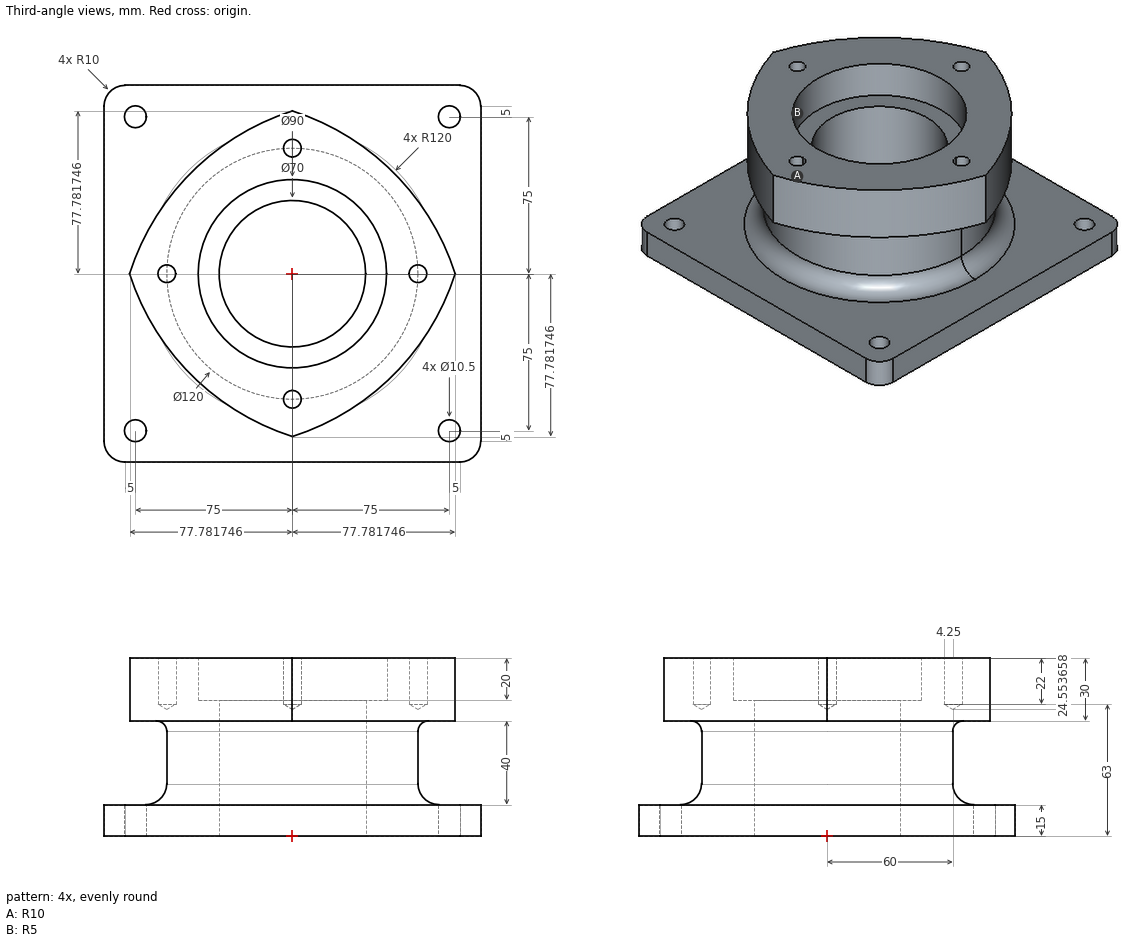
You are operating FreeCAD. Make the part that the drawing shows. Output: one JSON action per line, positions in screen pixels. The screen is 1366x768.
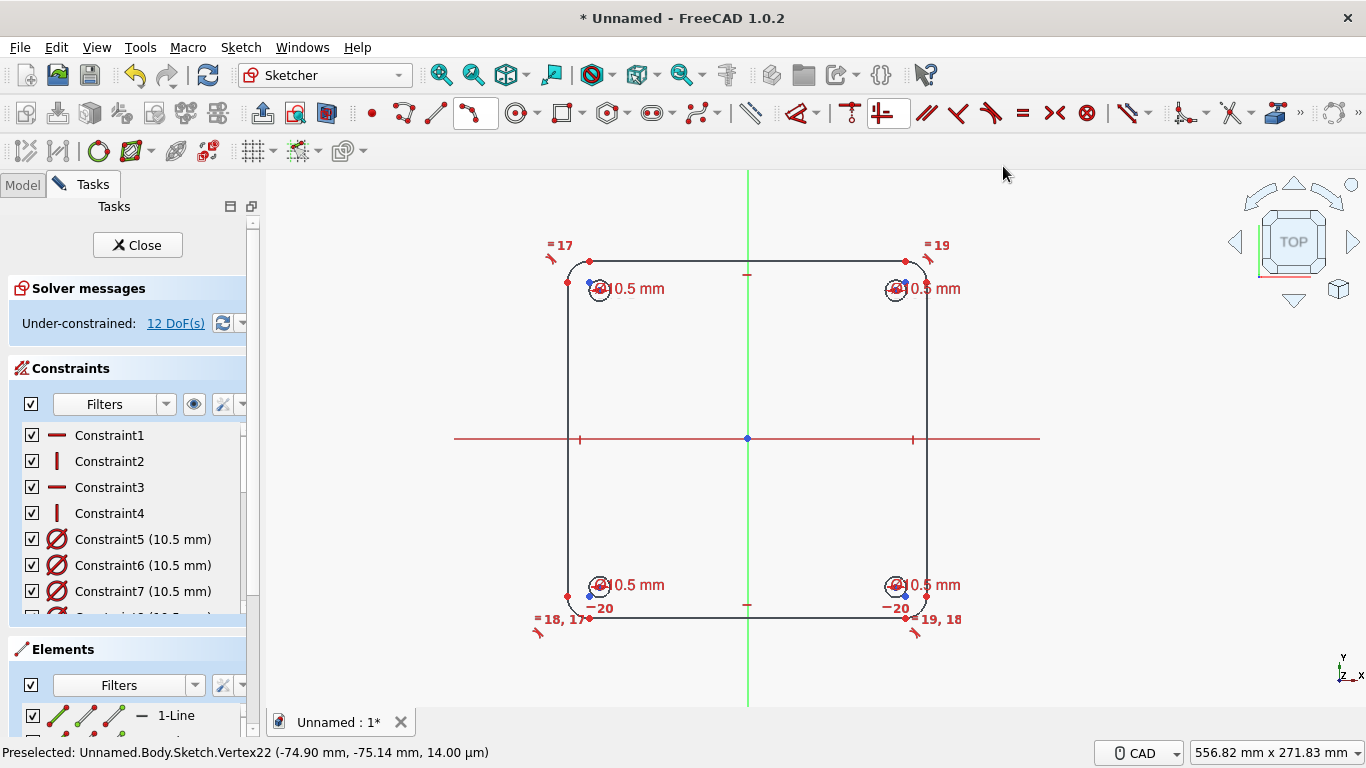
{"action": "left_click", "coordinate": [896, 587]}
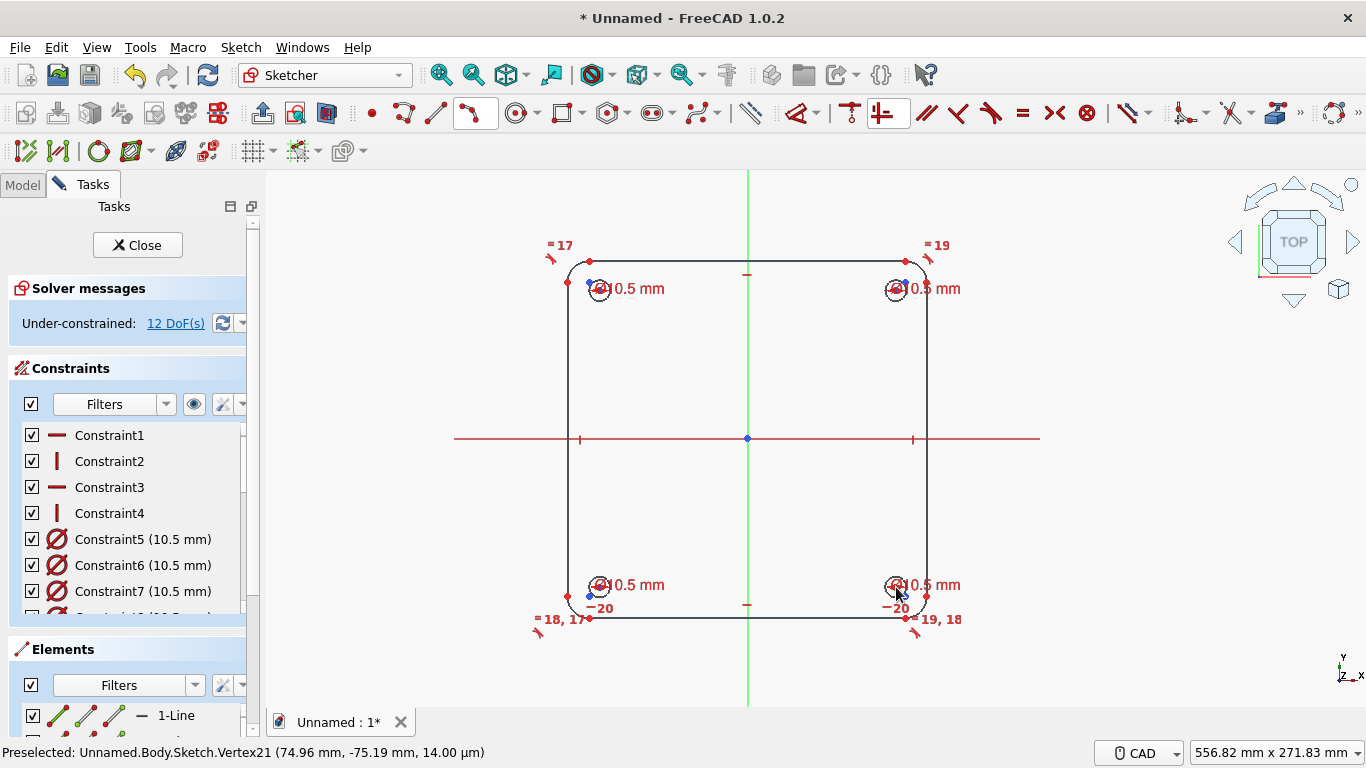
{"action": "left_click", "coordinate": [896, 291]}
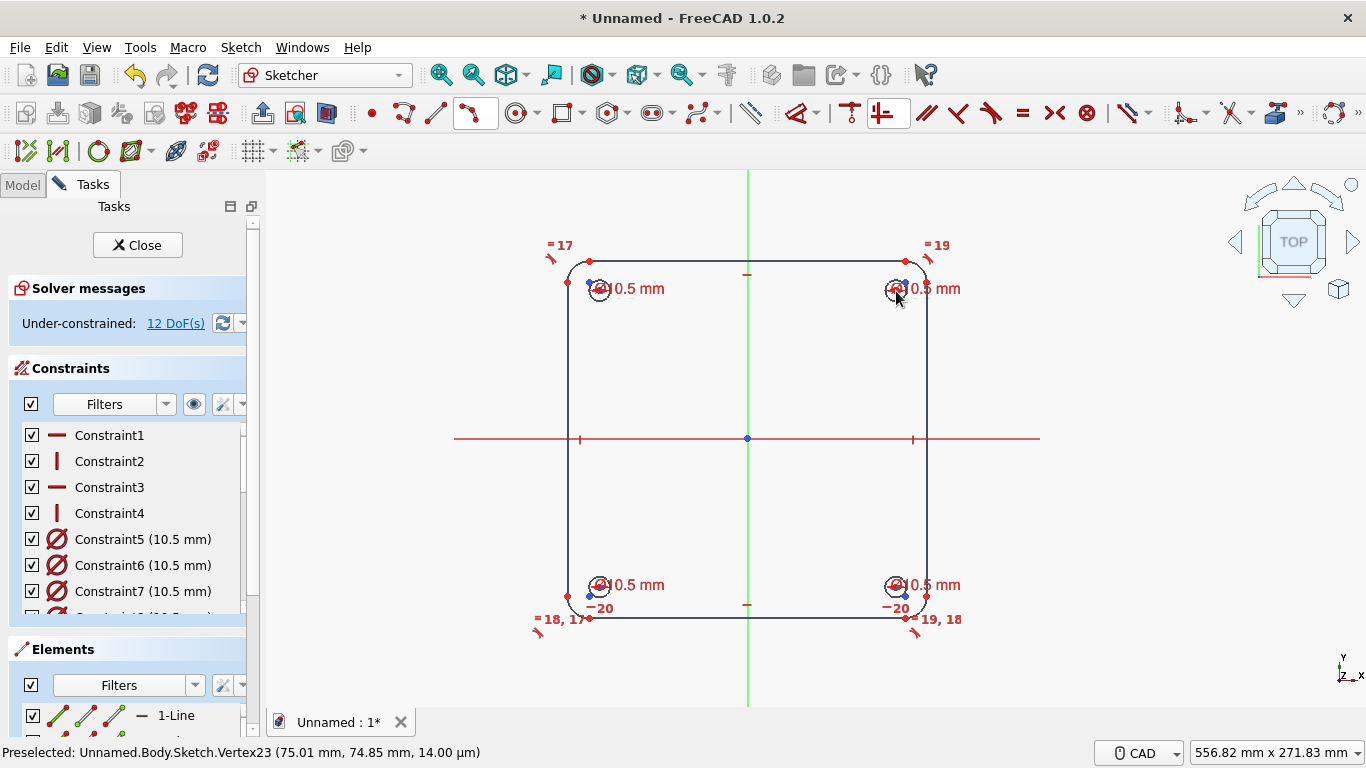
{"action": "left_click", "coordinate": [904, 114]}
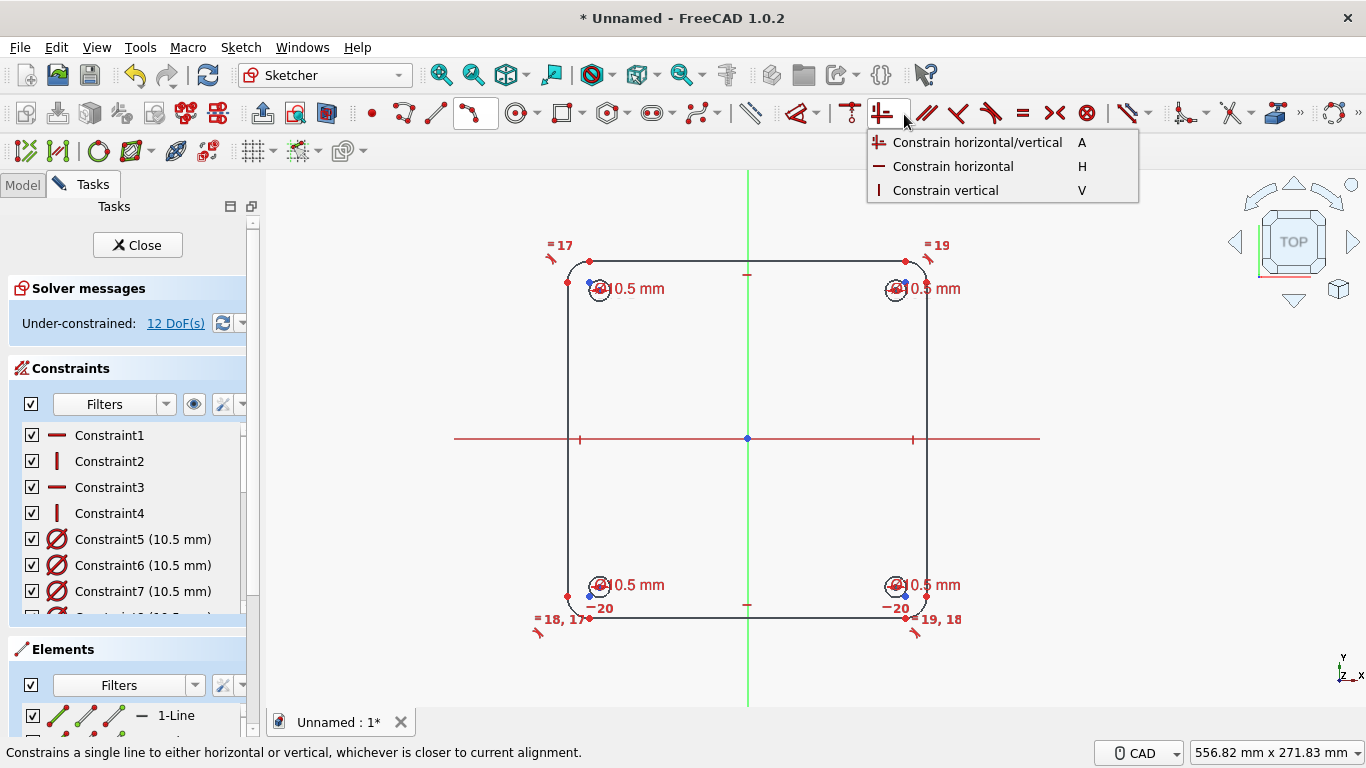
{"action": "left_click", "coordinate": [1003, 190]}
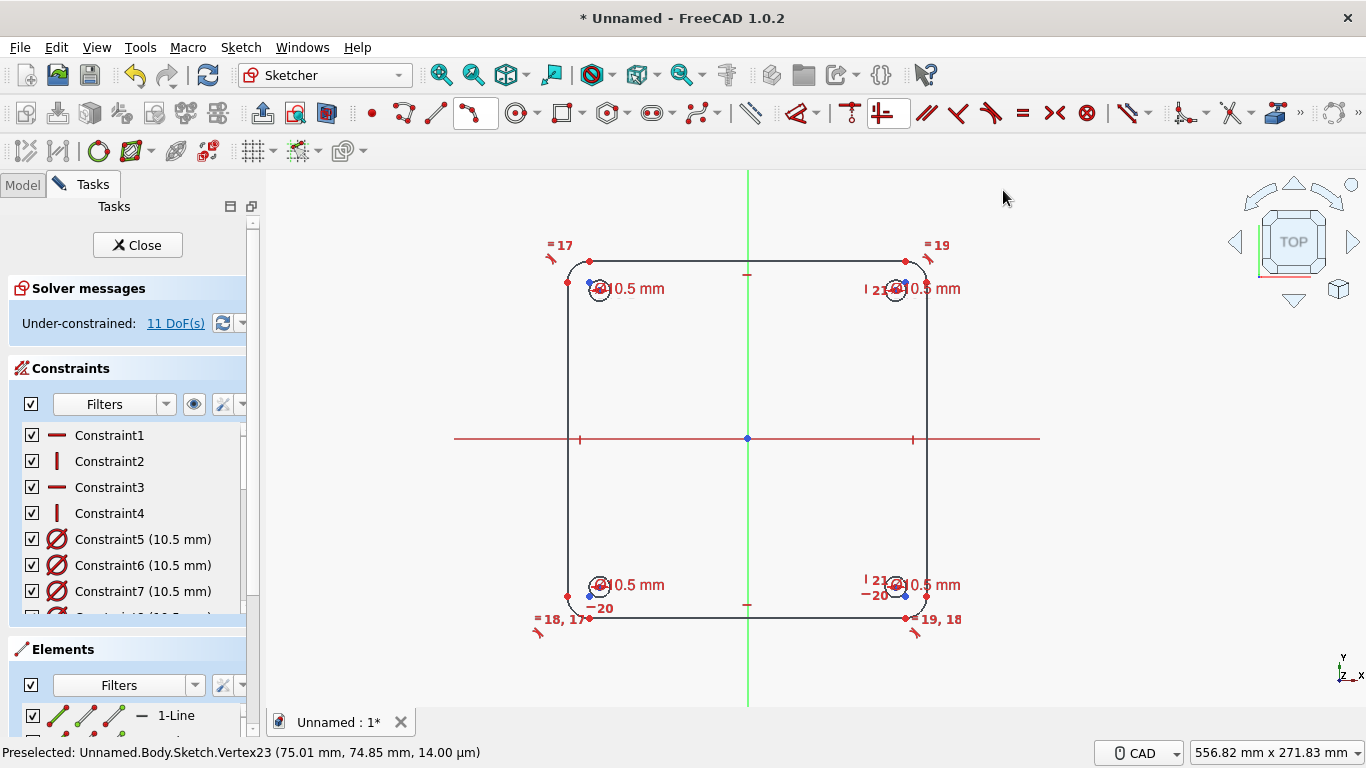
{"action": "left_click", "coordinate": [600, 587]}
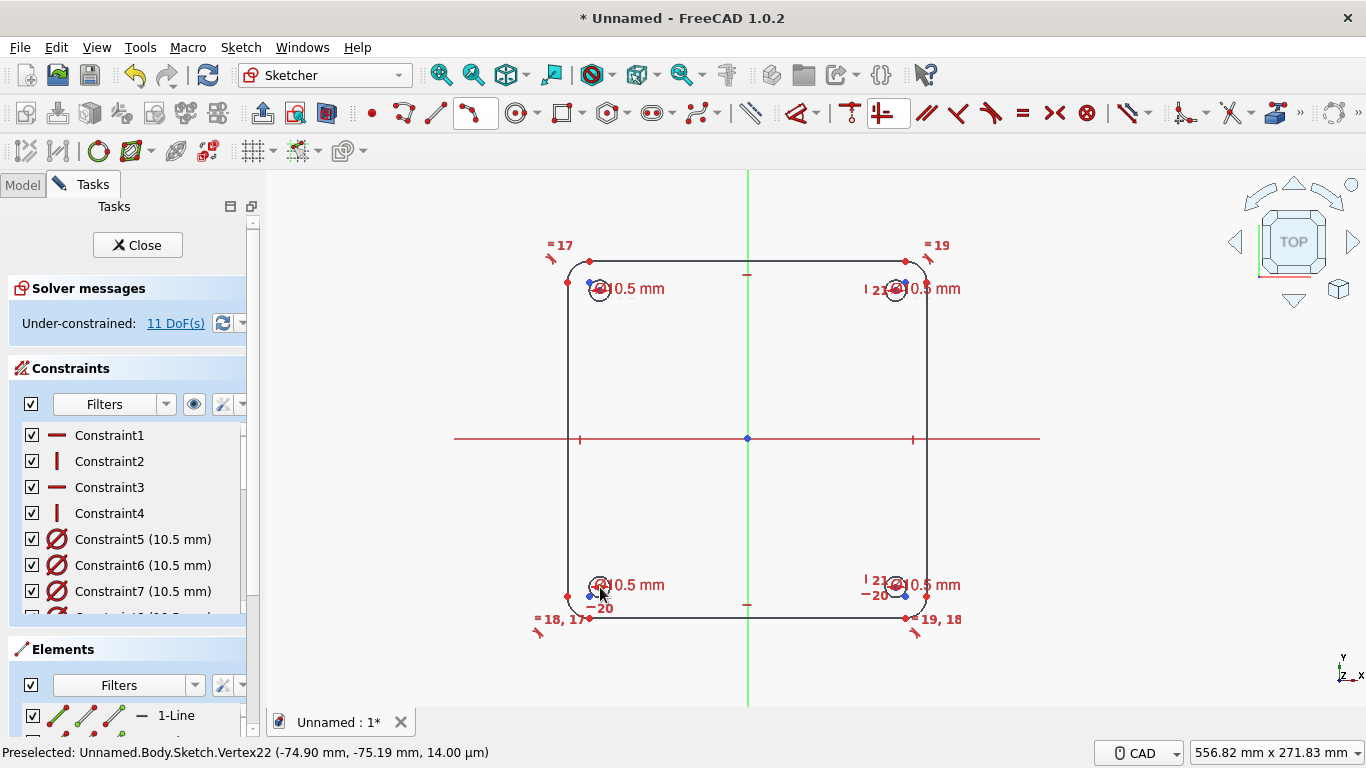
{"action": "left_click", "coordinate": [600, 291]}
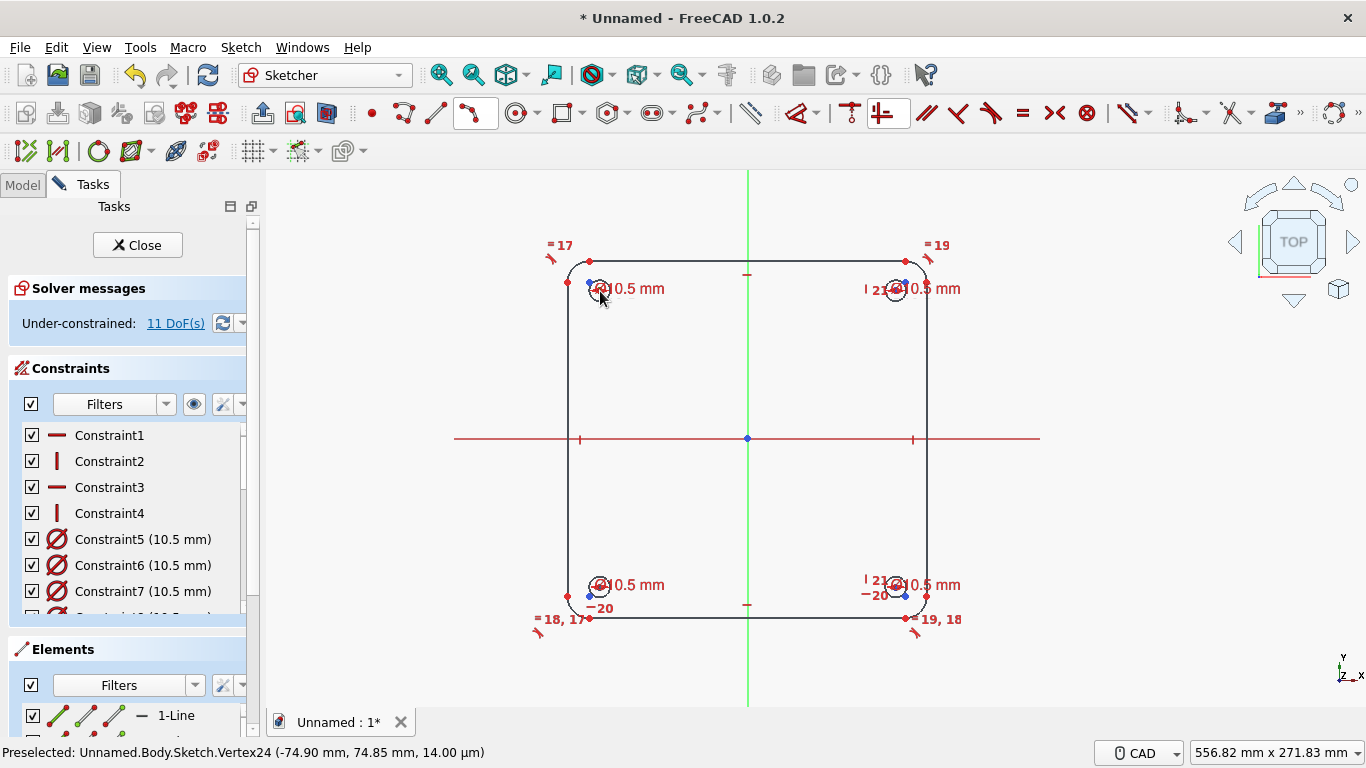
{"action": "left_click", "coordinate": [904, 114]}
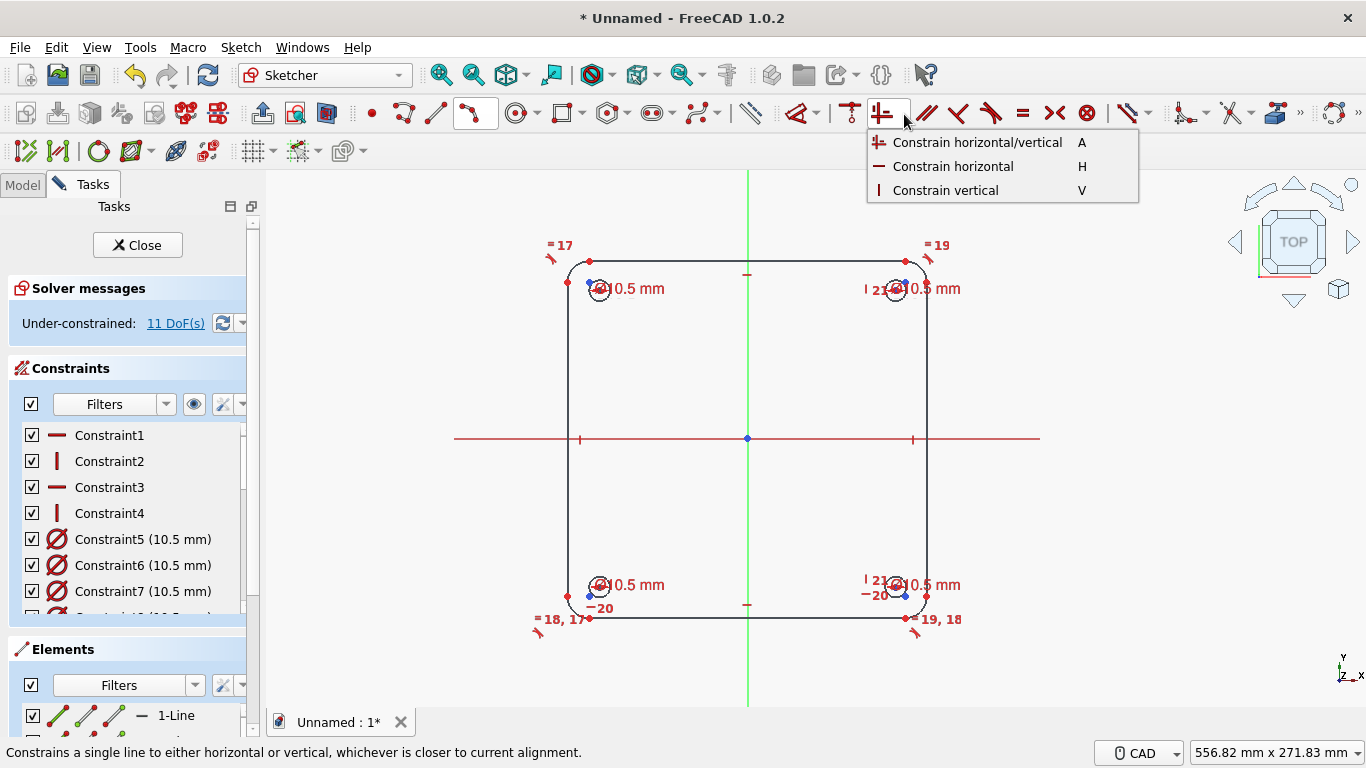
{"action": "left_click", "coordinate": [1003, 190]}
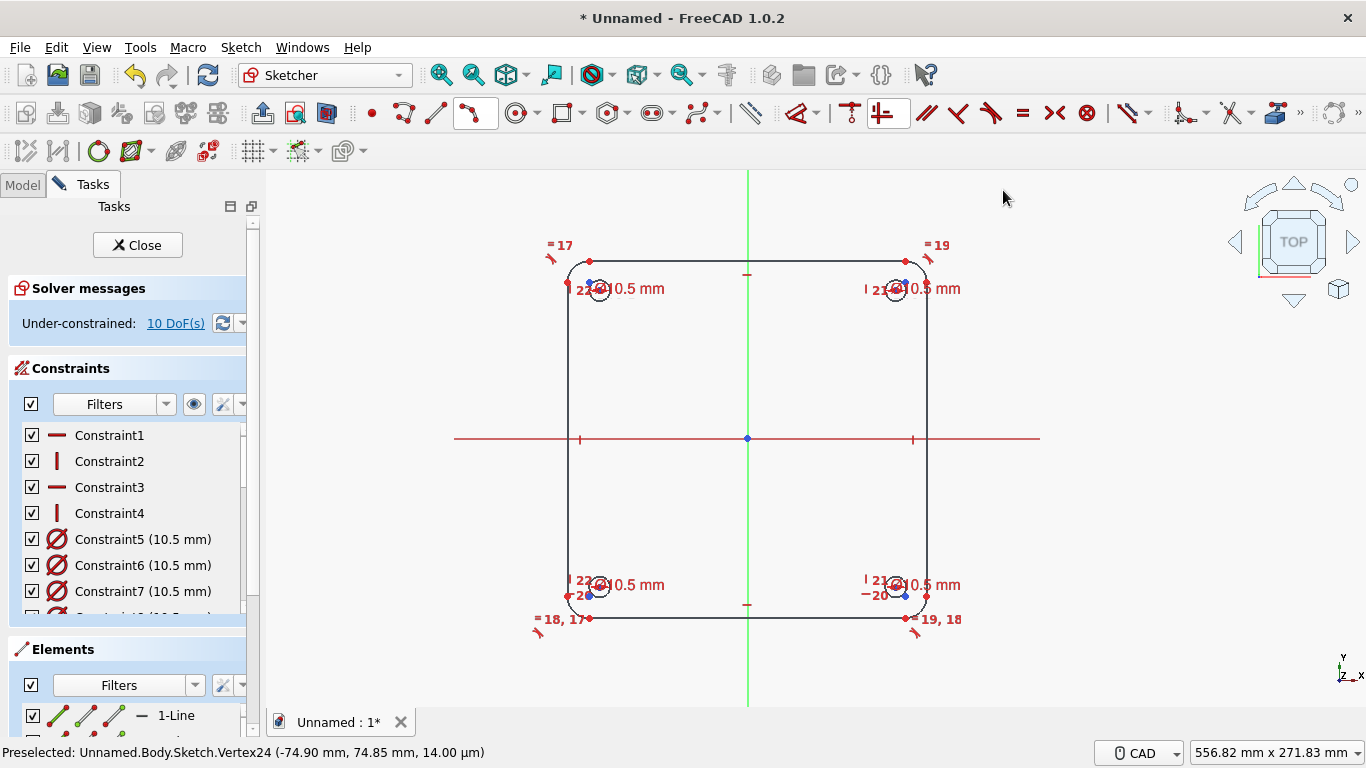
{"action": "left_click", "coordinate": [896, 291]}